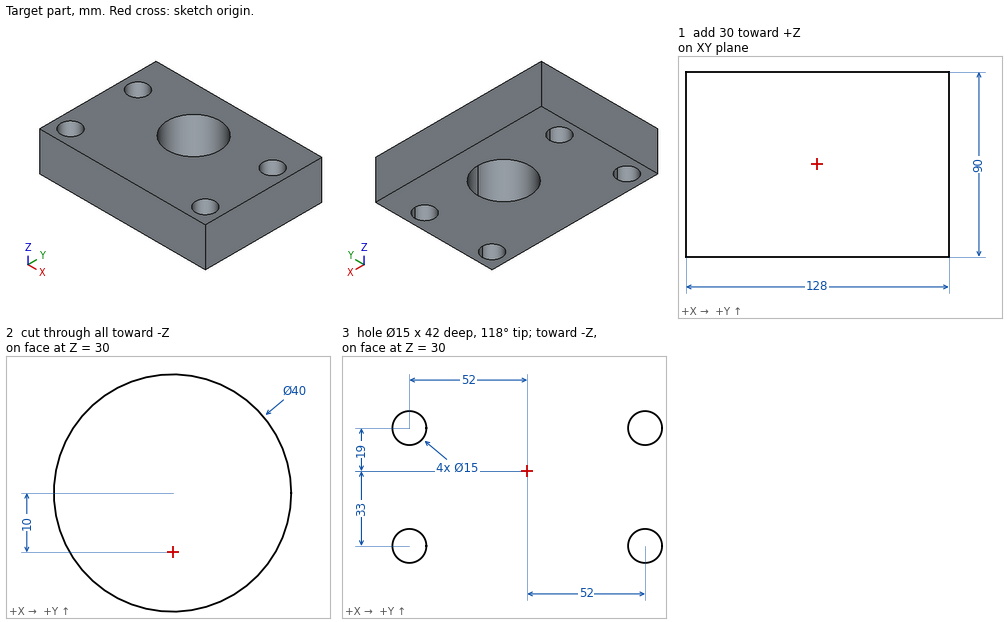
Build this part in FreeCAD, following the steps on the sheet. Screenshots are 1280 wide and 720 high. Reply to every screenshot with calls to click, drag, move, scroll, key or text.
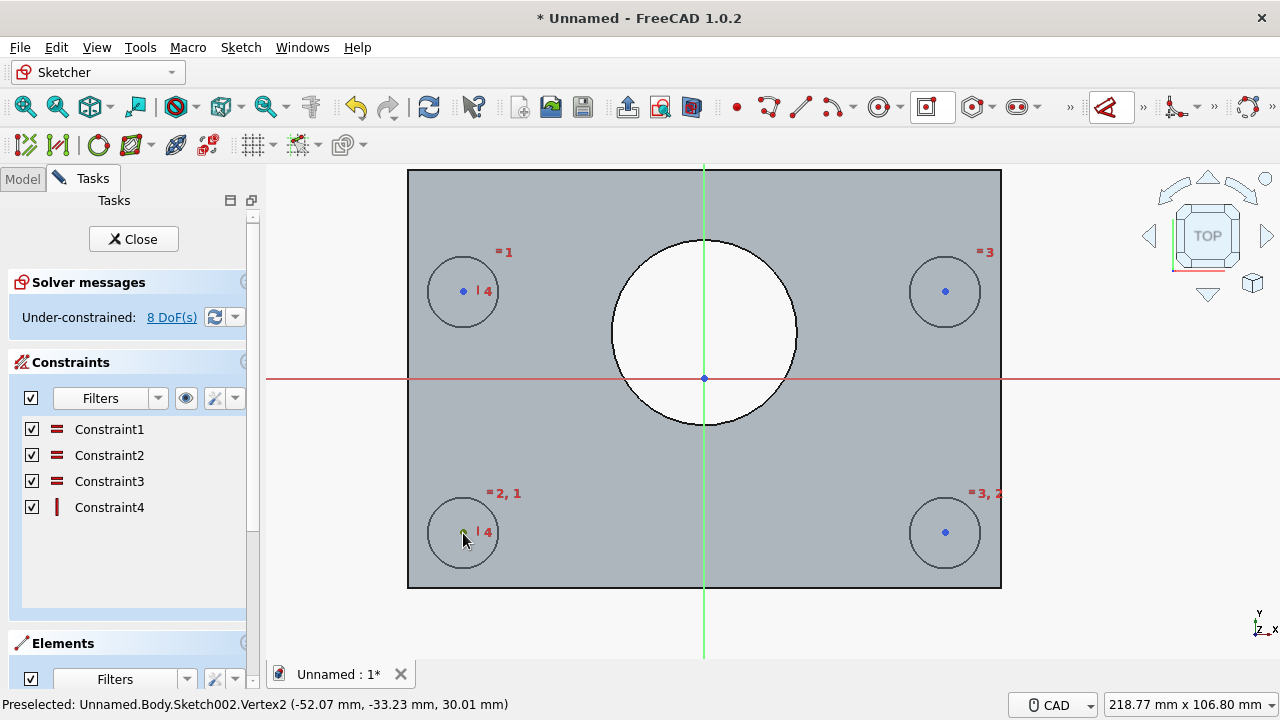
click(945, 533)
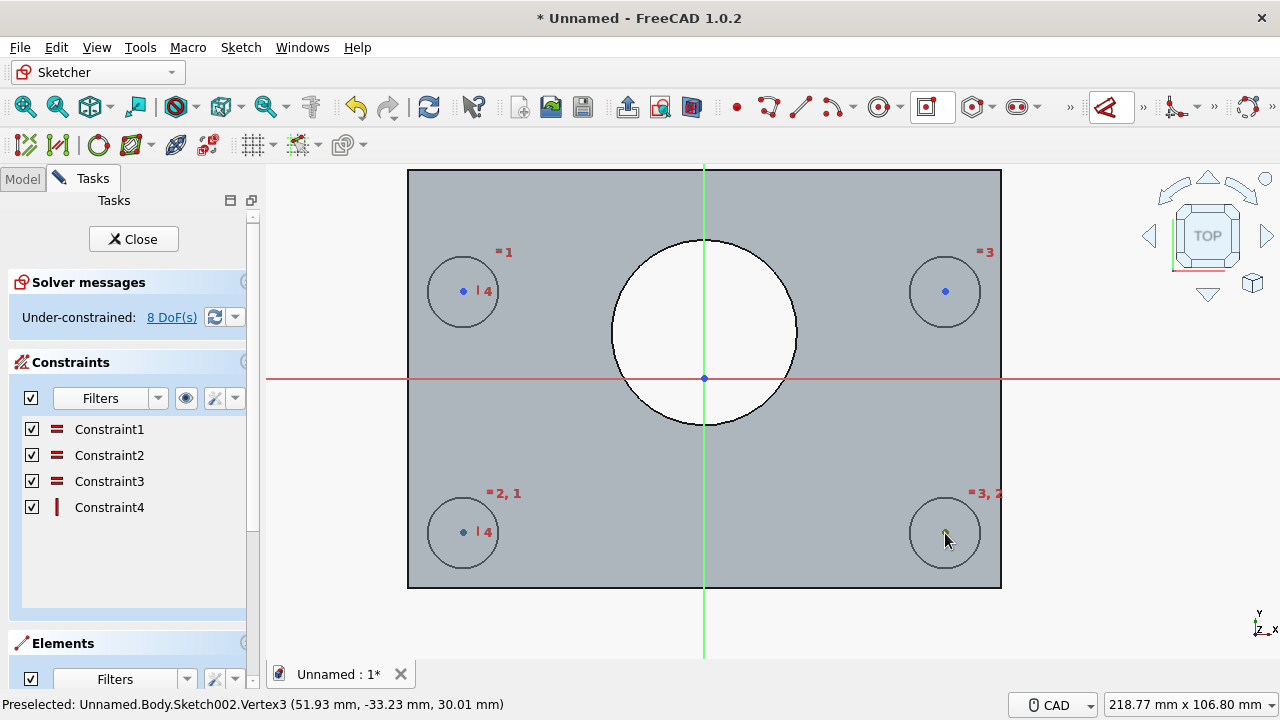
key(h)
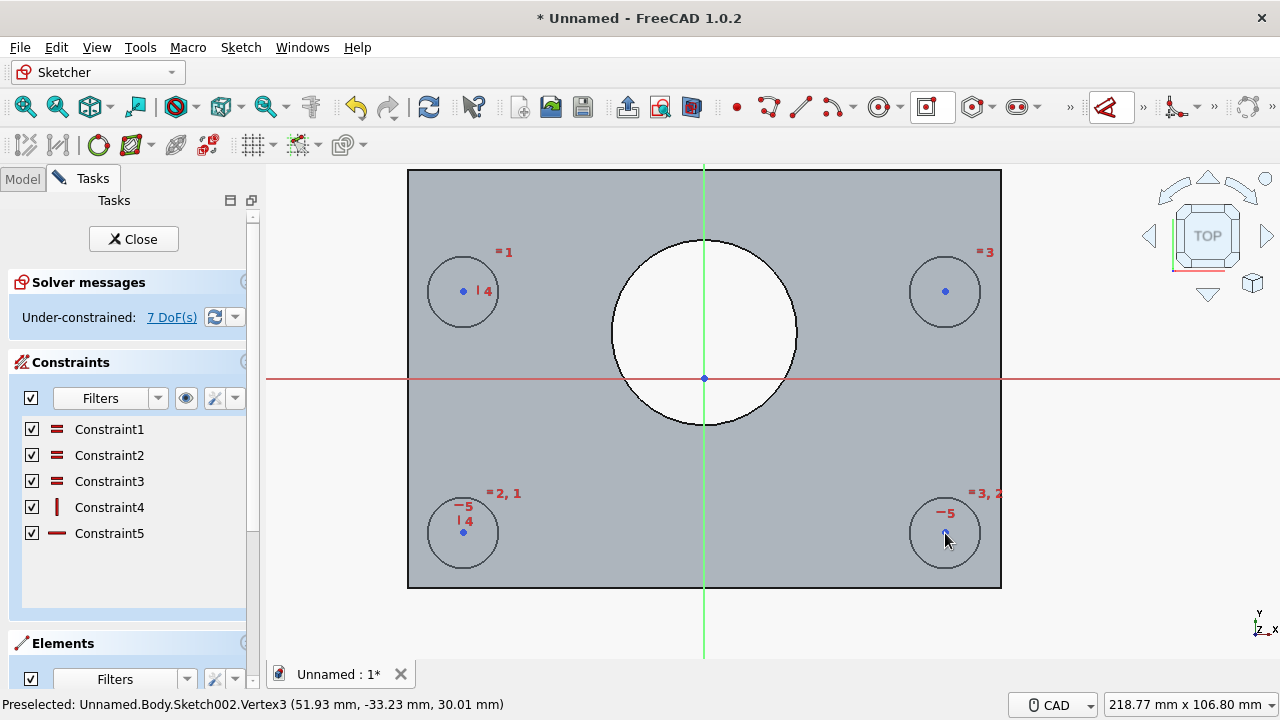
click(945, 533)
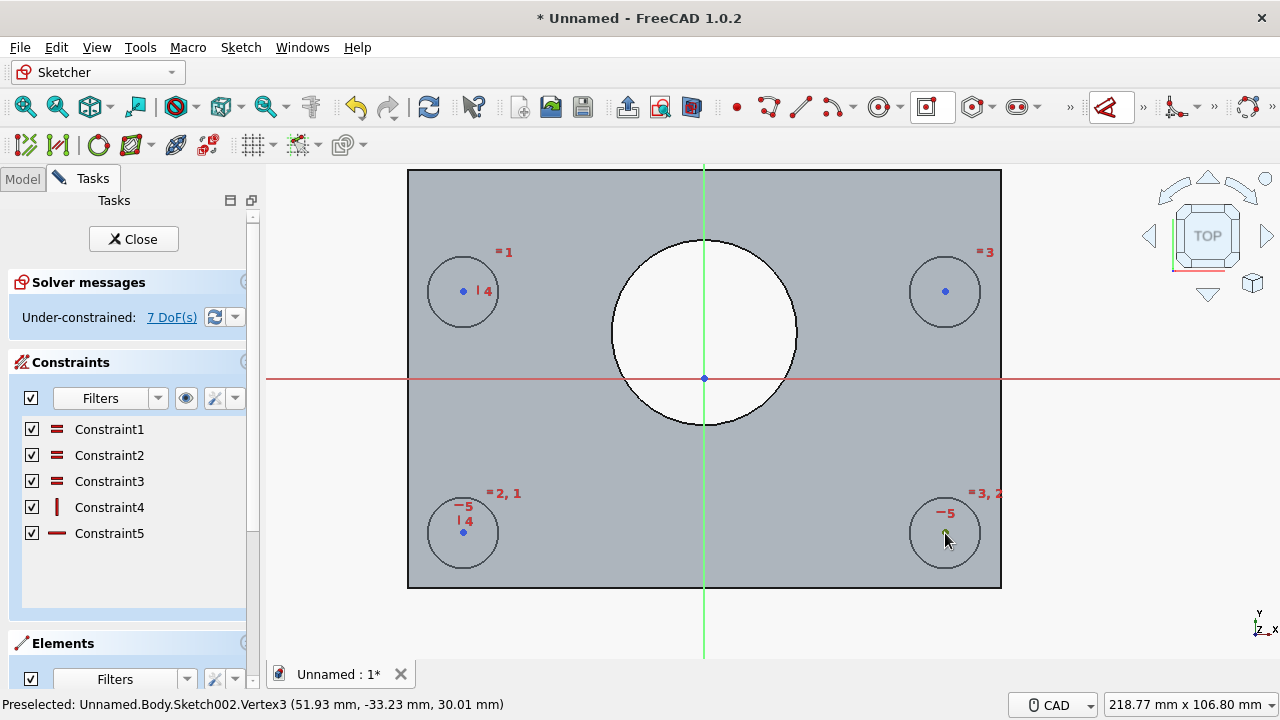
click(945, 292)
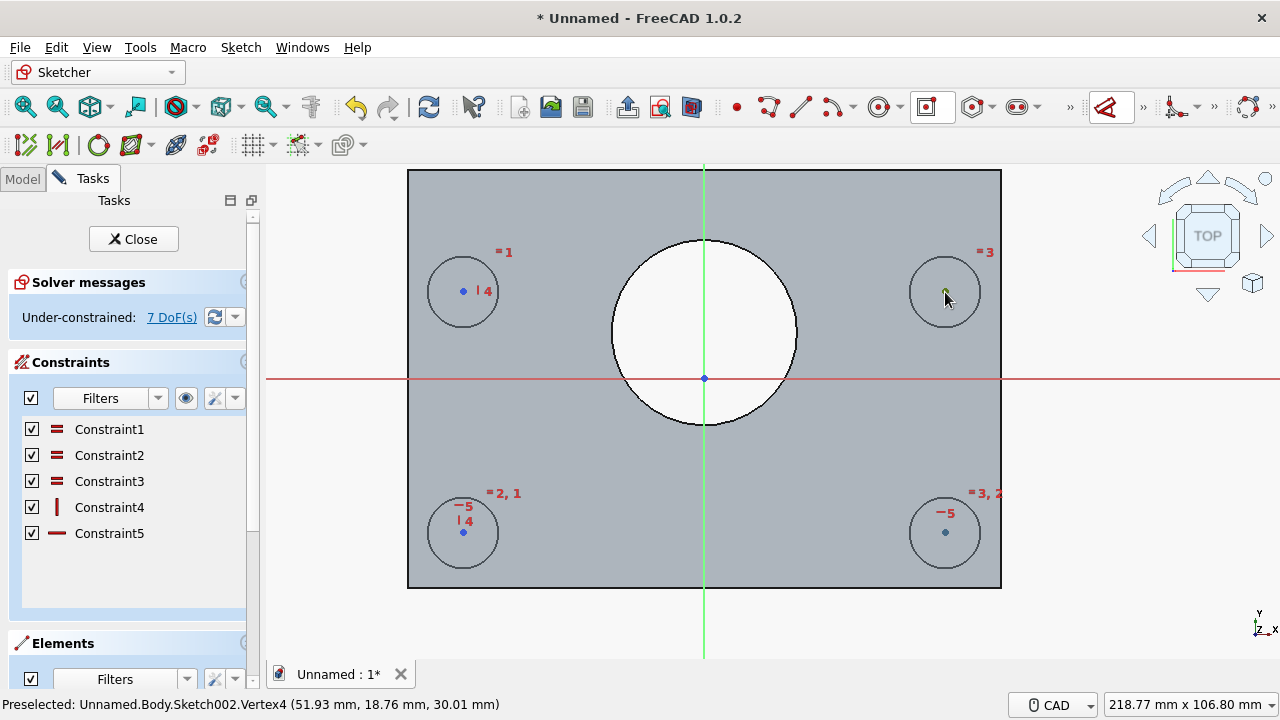
key(v)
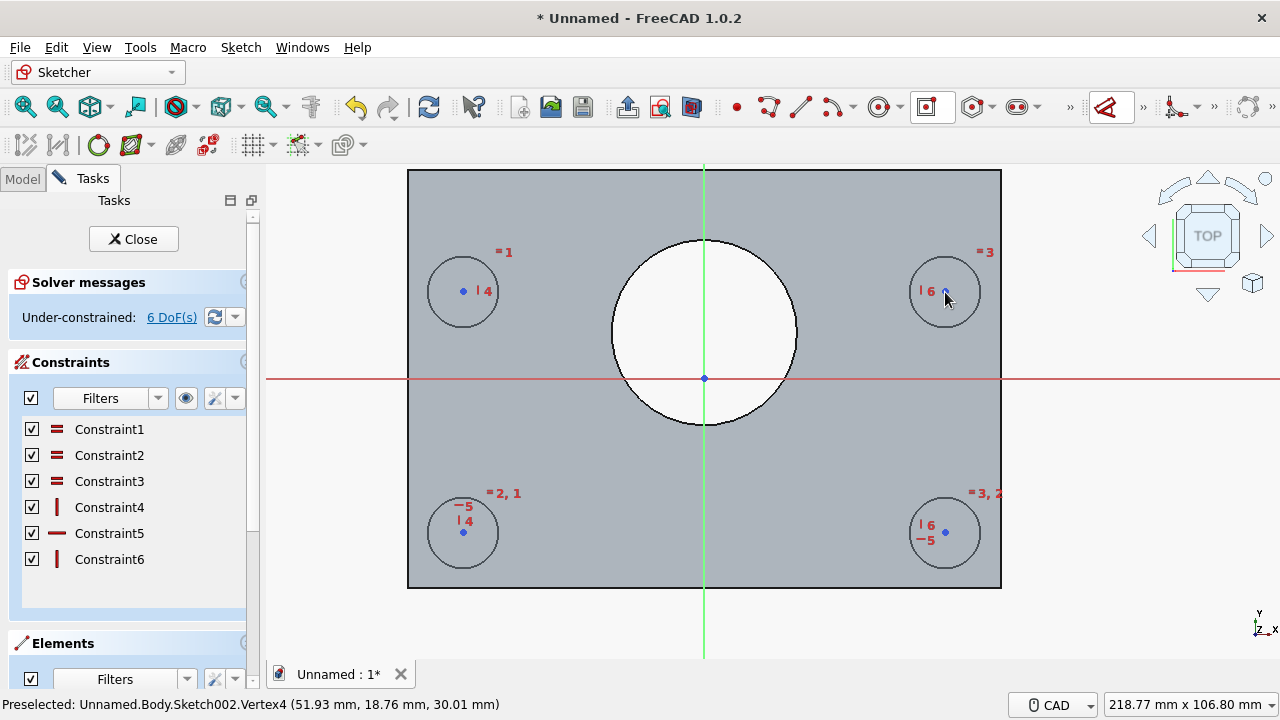
click(463, 292)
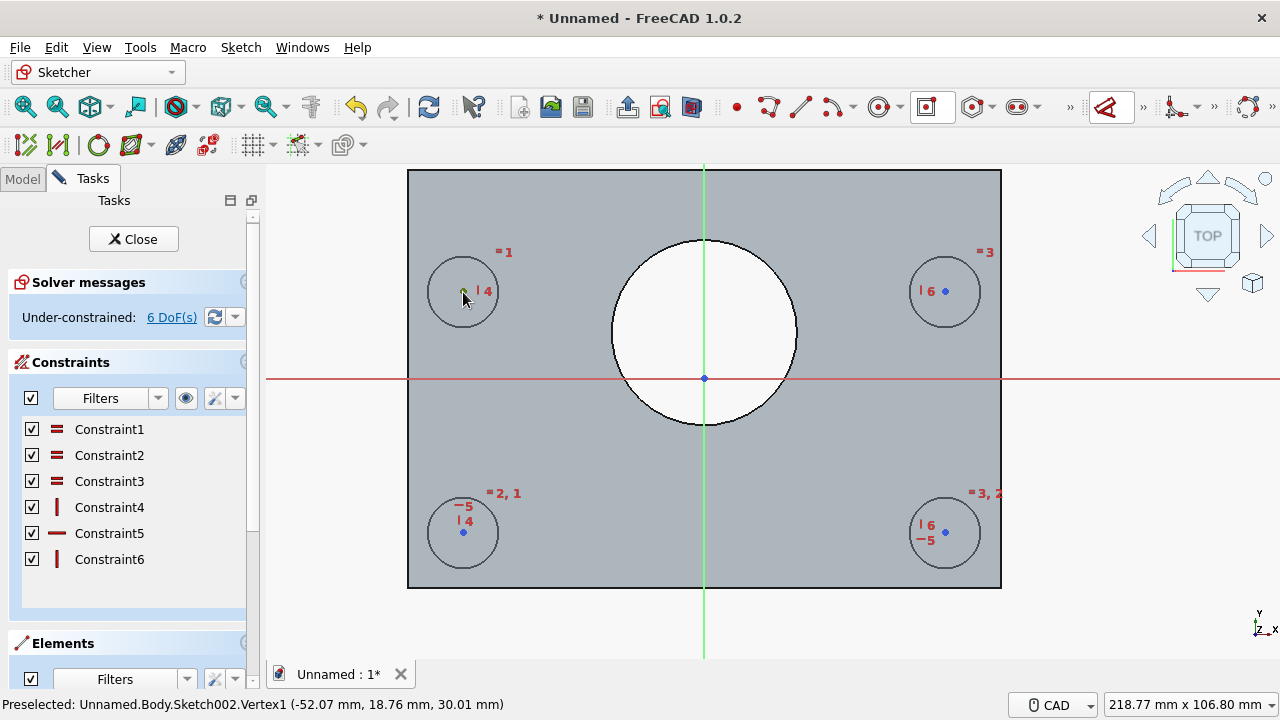
click(945, 292)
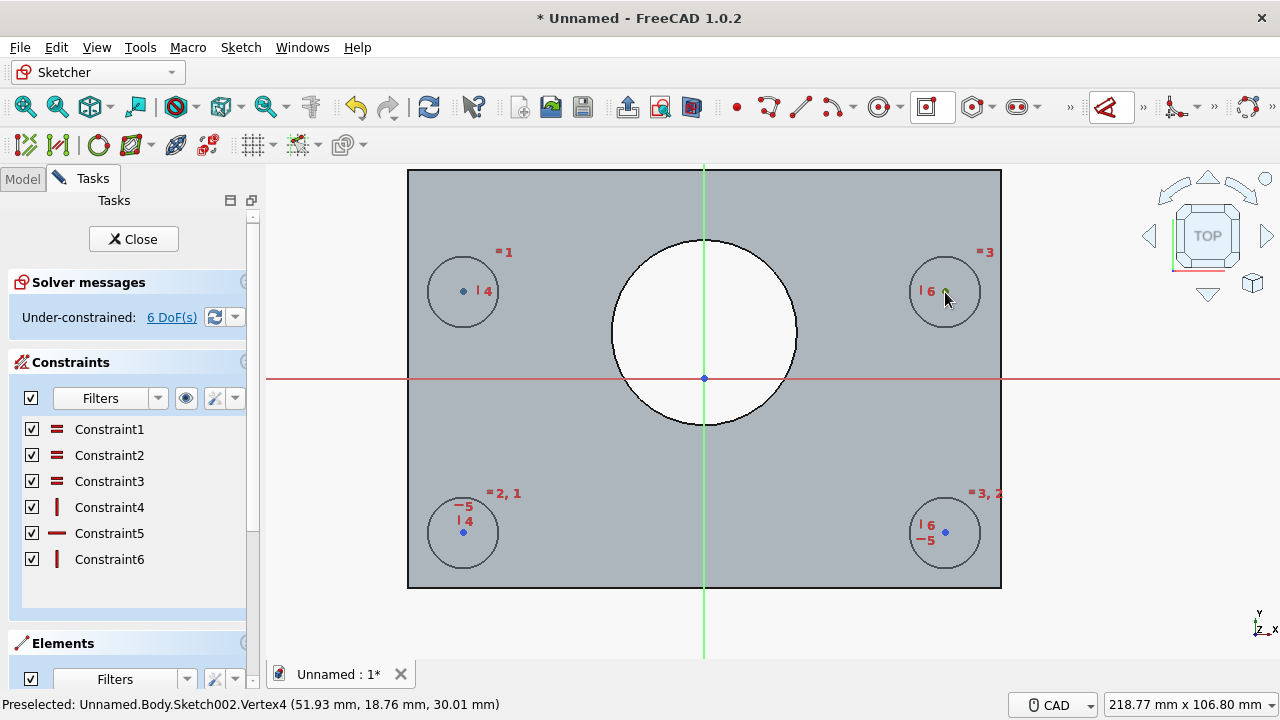
key(h)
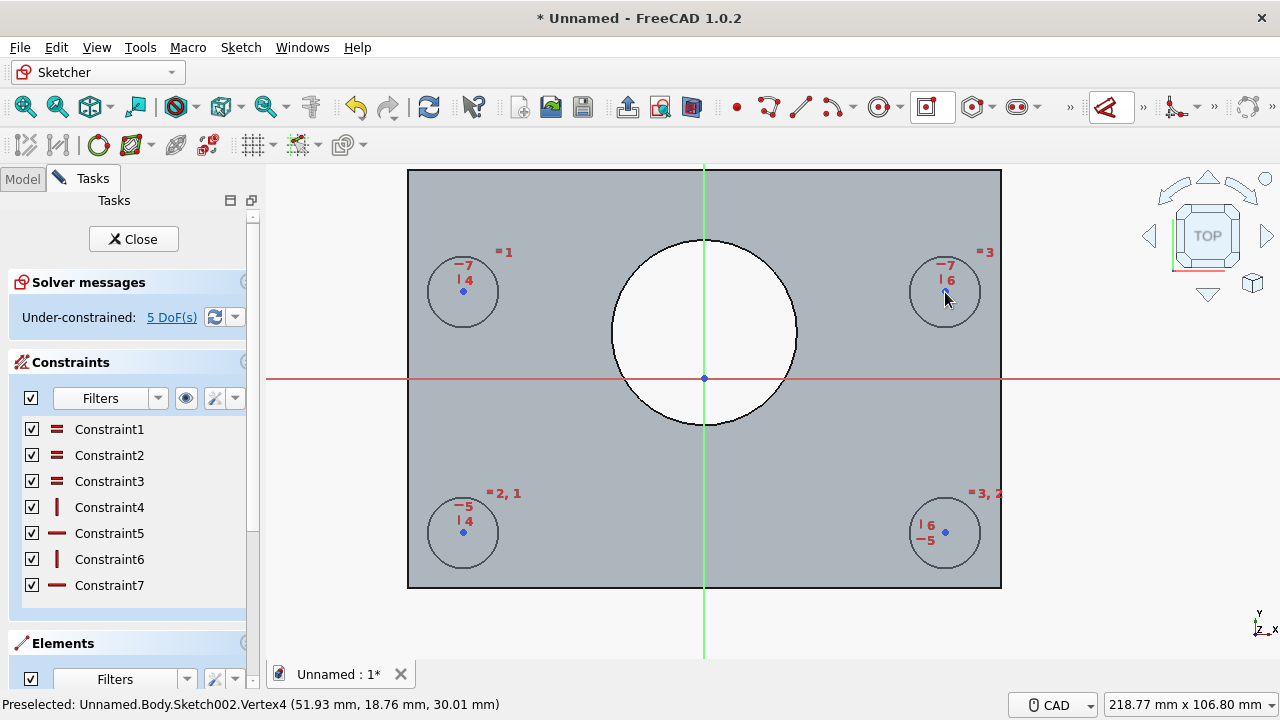
click(488, 267)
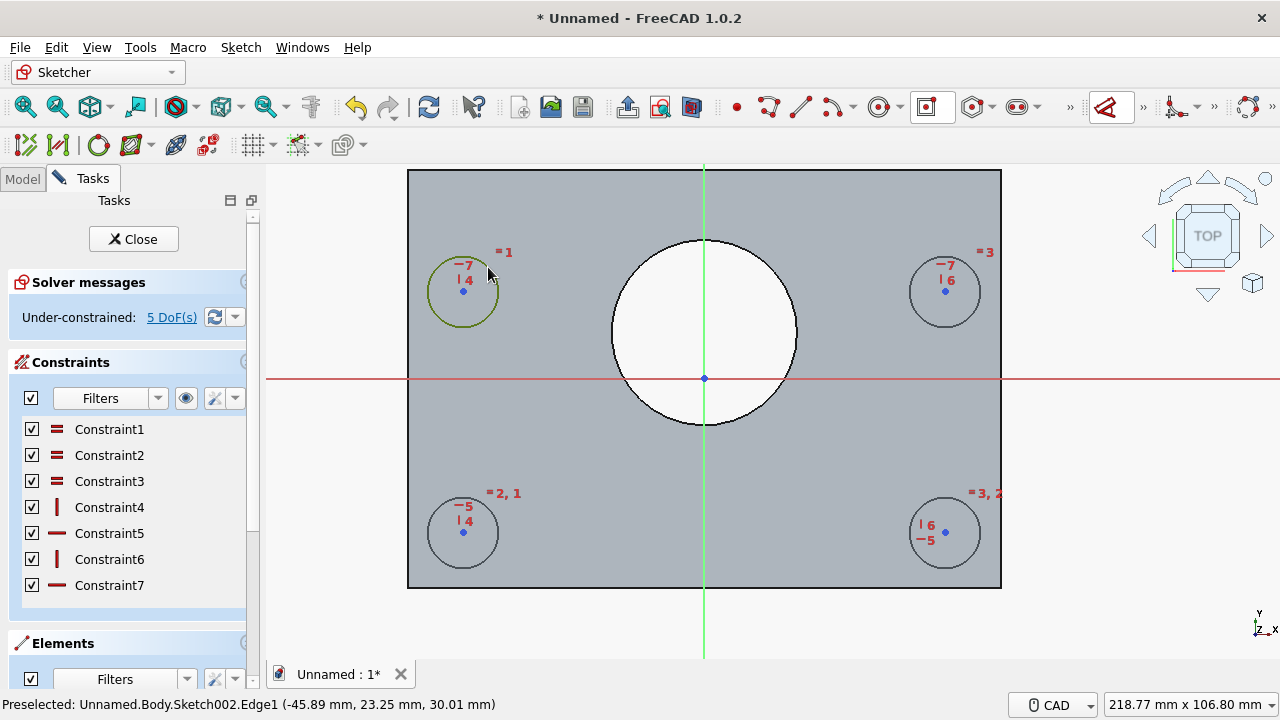
key(k)
key(o)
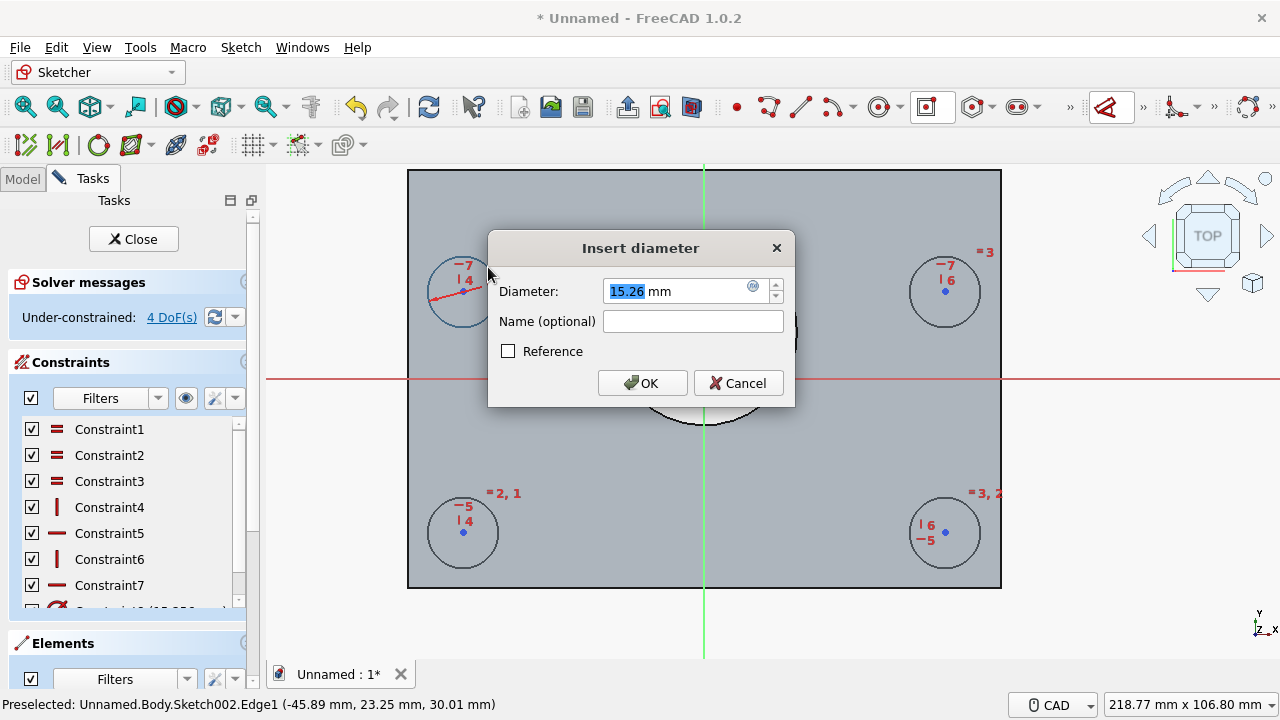
text(15)
key(Return)